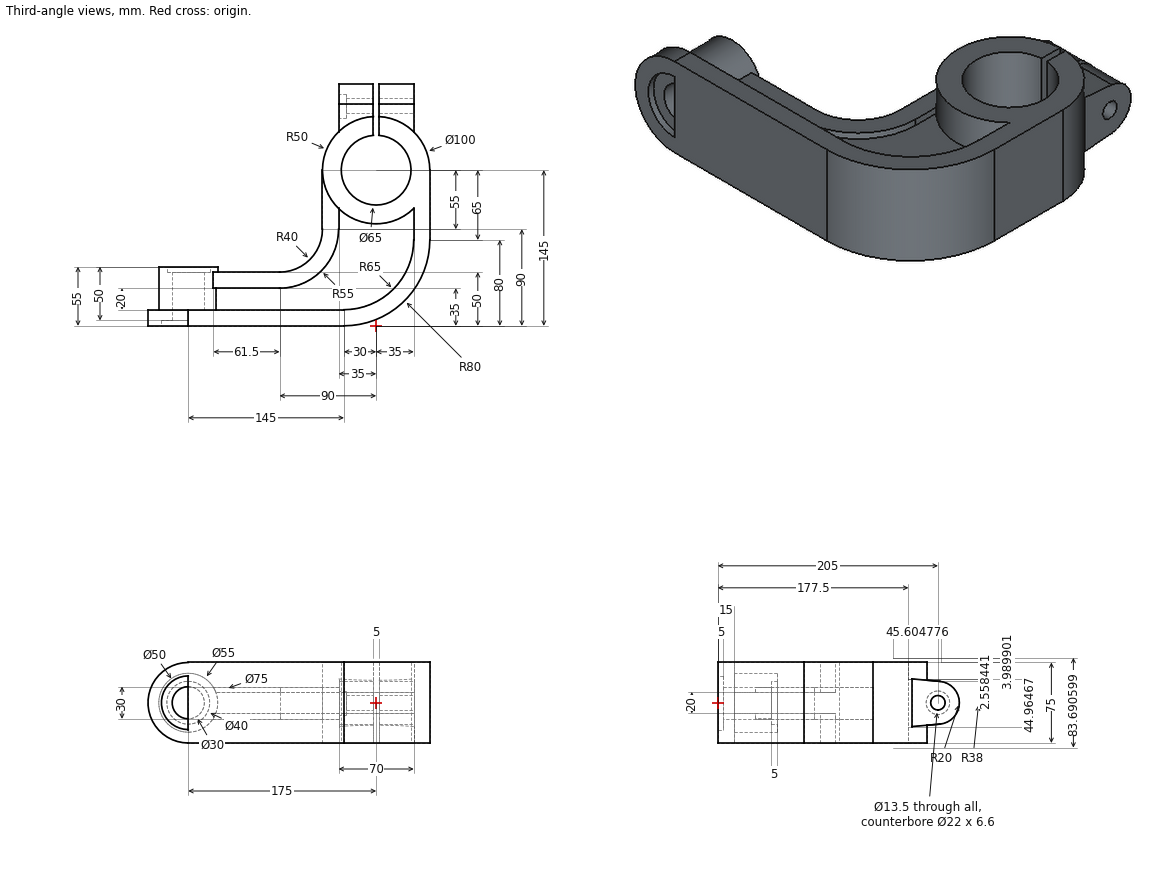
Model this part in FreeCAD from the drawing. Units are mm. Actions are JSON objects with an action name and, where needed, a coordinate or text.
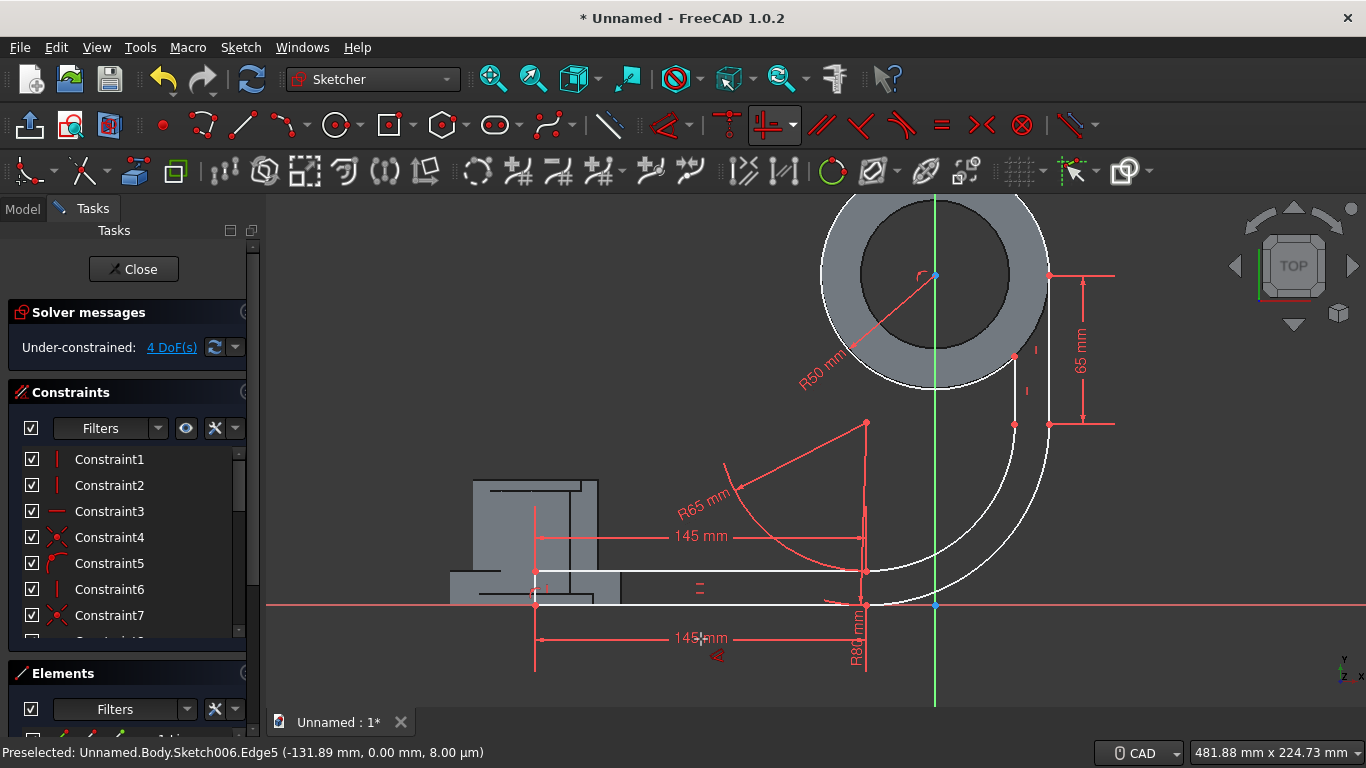
{"action": "left_click", "coordinate": [1049, 424]}
{"action": "left_click", "coordinate": [1083, 515]}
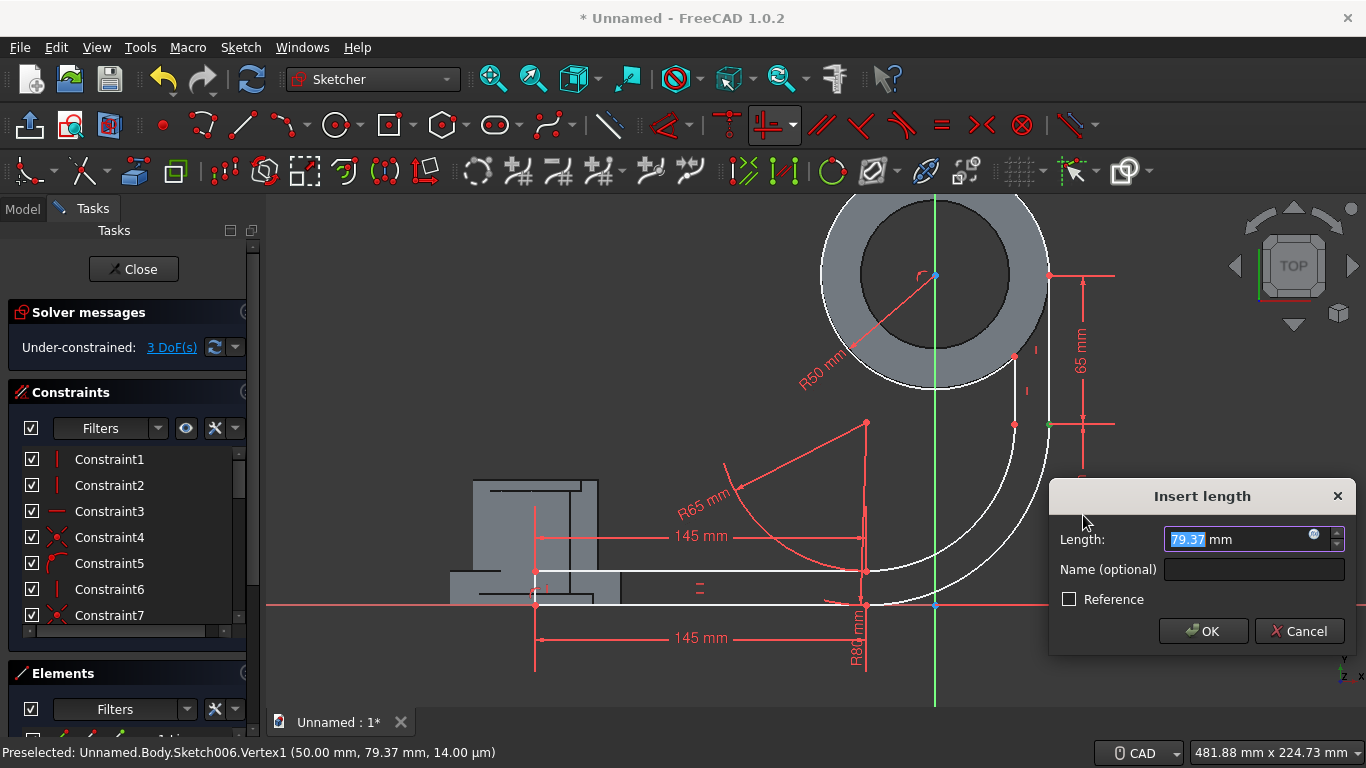
{"action": "type", "text": "80"}
{"action": "key", "text": "Return"}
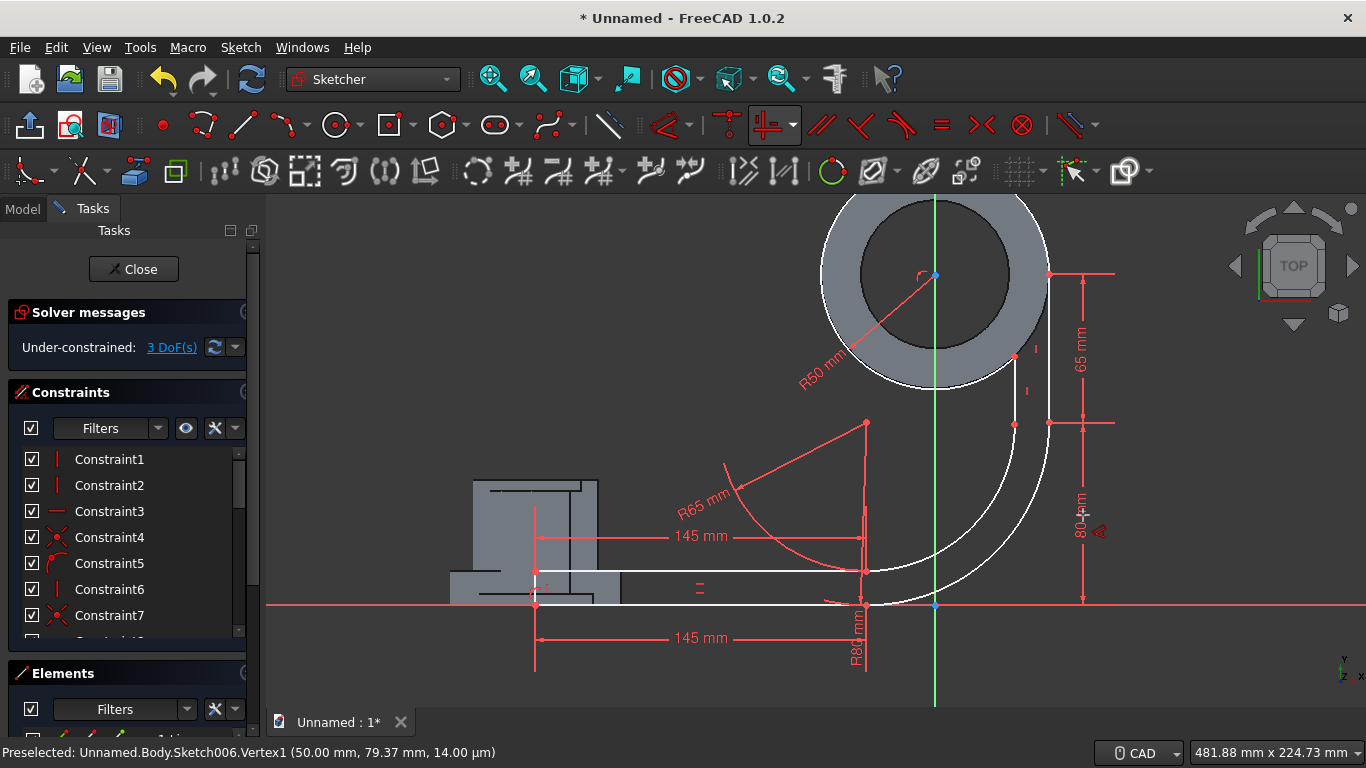
{"action": "left_click", "coordinate": [1015, 424]}
{"action": "left_click", "coordinate": [1049, 556]}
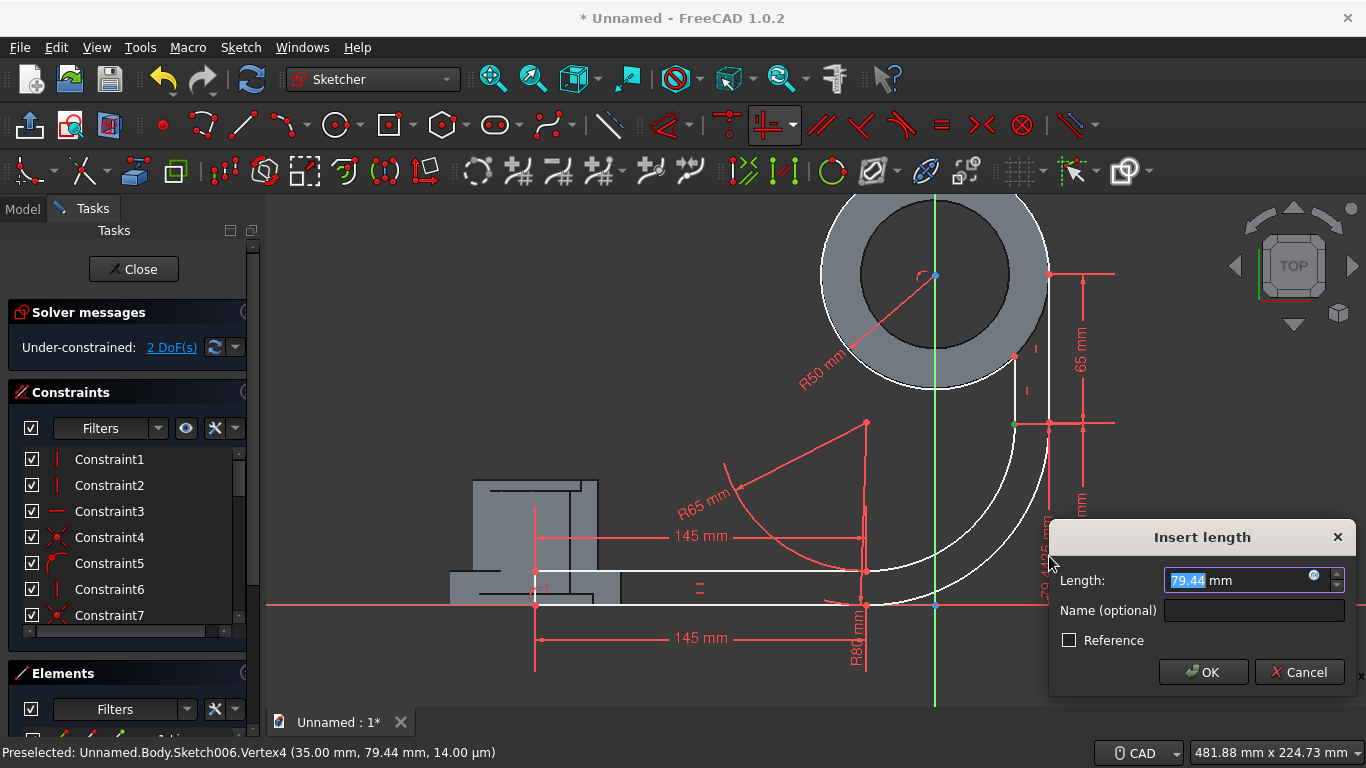
{"action": "type", "text": "80"}
{"action": "key", "text": "Return"}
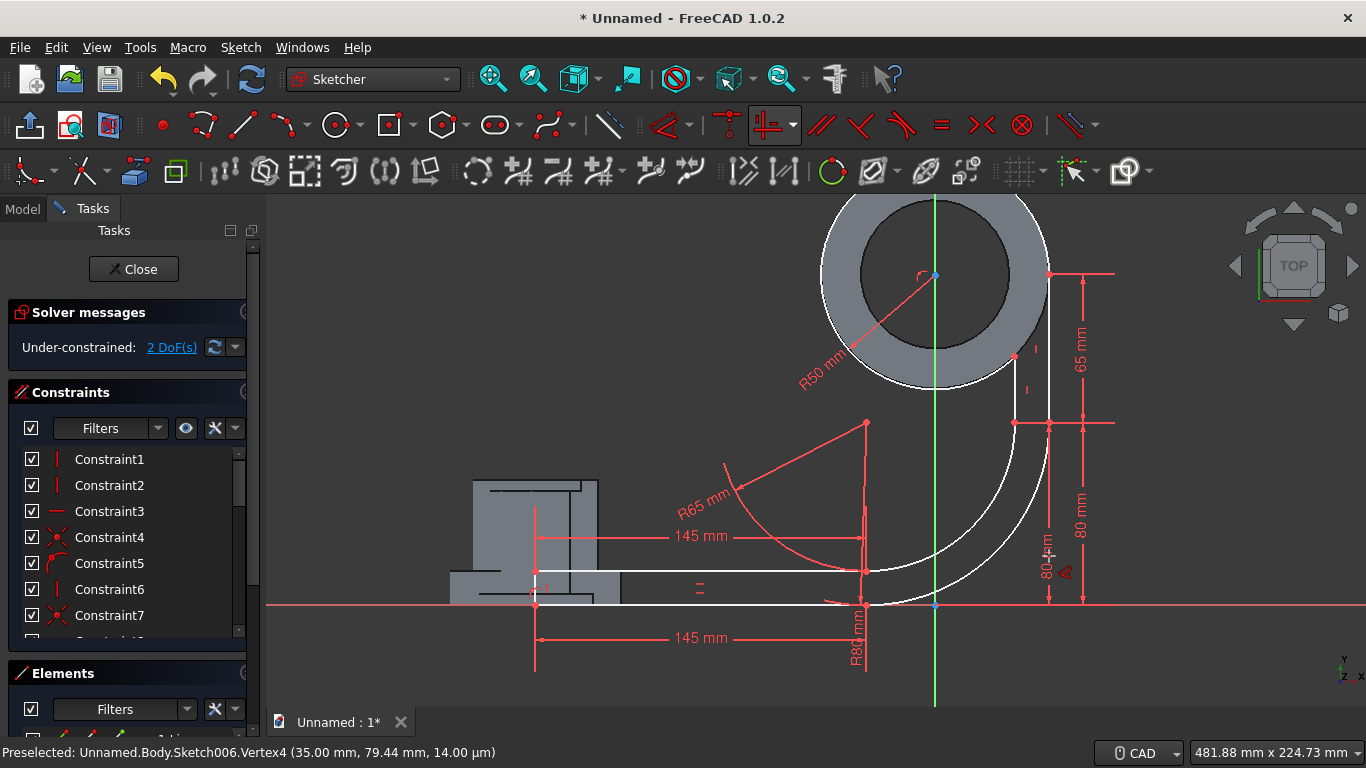
{"action": "left_click", "coordinate": [866, 571]}
{"action": "left_click", "coordinate": [901, 537]}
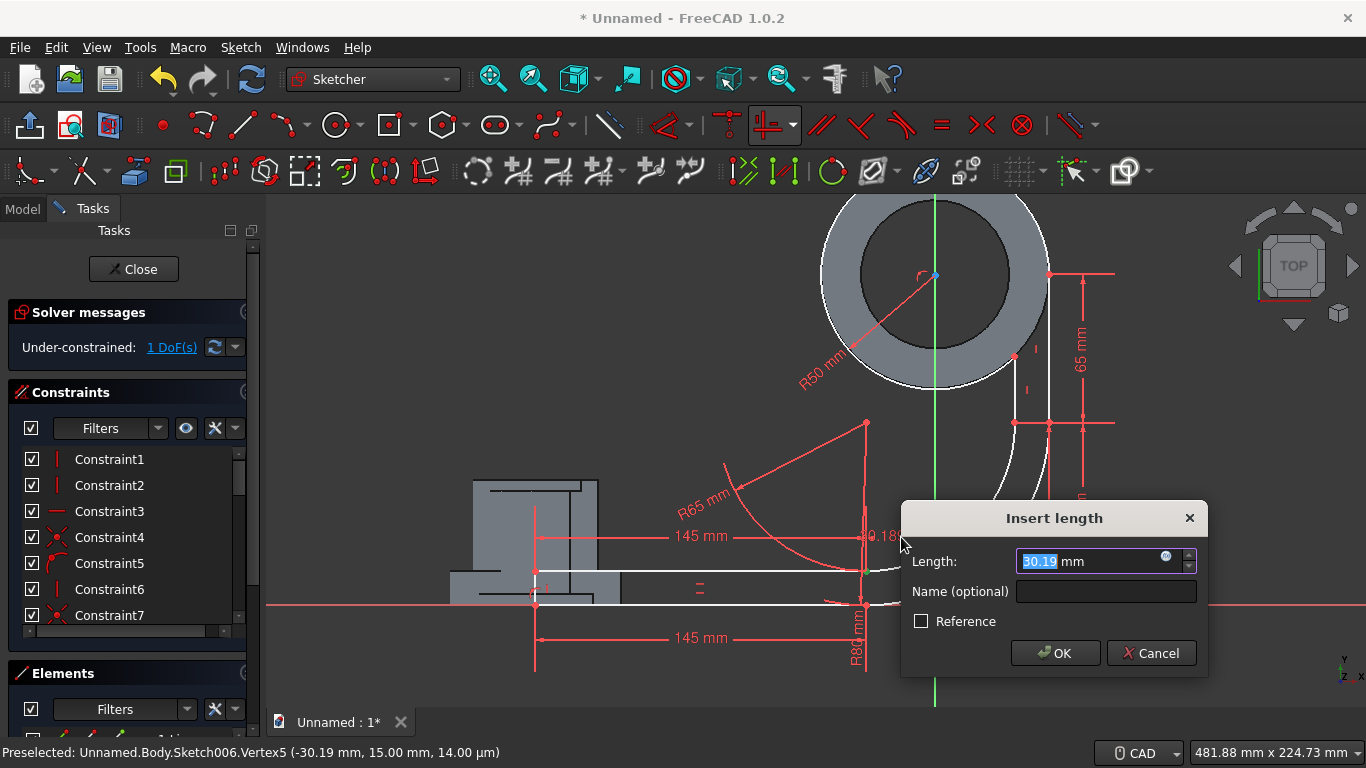
{"action": "type", "text": "30"}
{"action": "key", "text": "Return"}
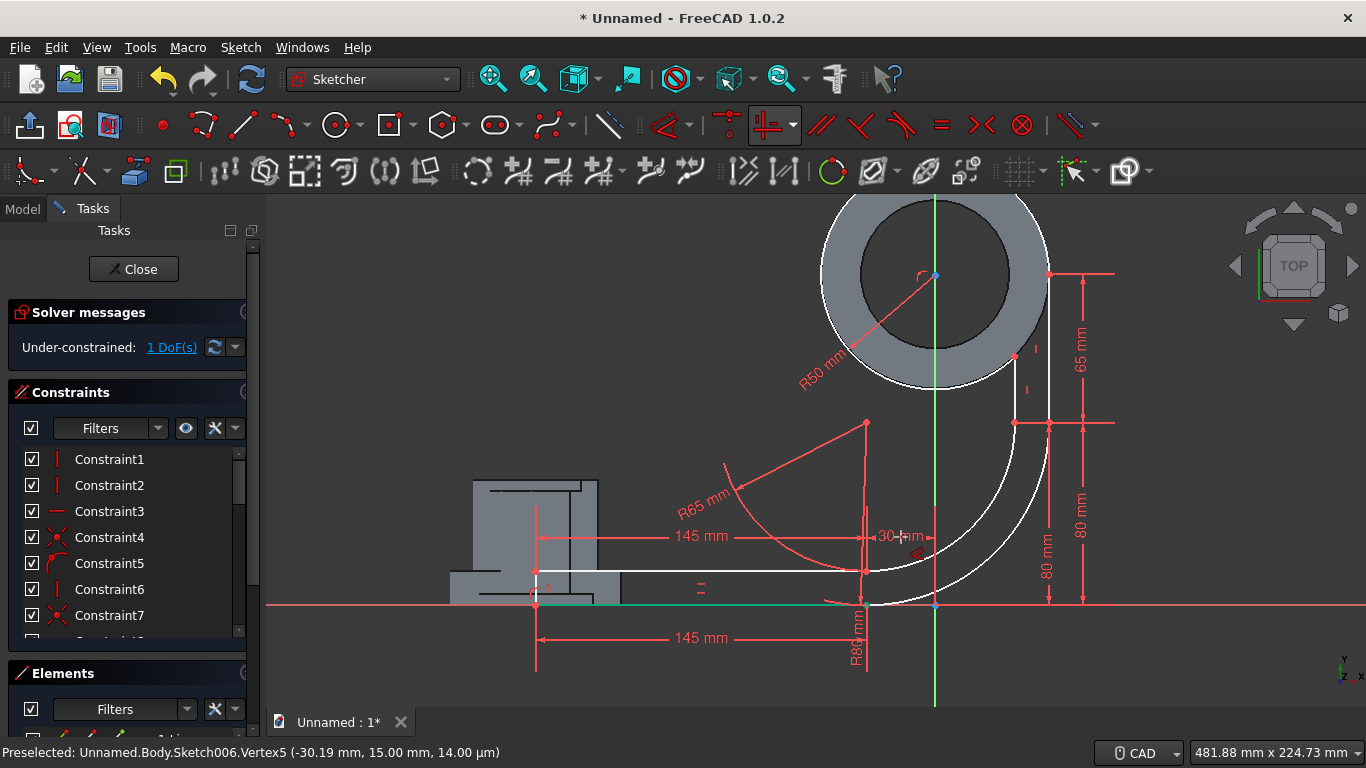
{"action": "left_click", "coordinate": [935, 275]}
{"action": "left_click", "coordinate": [969, 440]}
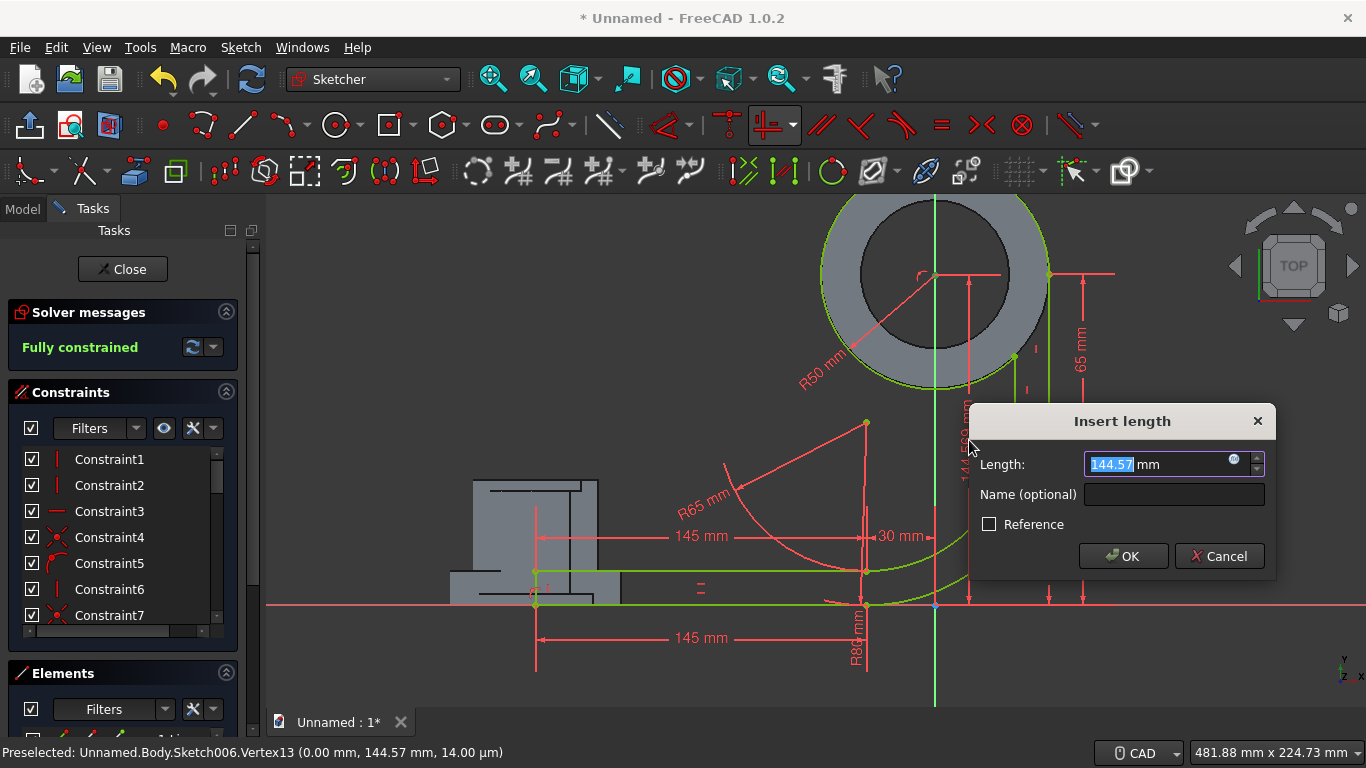
{"action": "type", "text": "145"}
{"action": "key", "text": "Return"}
{"action": "key", "text": "Escape"}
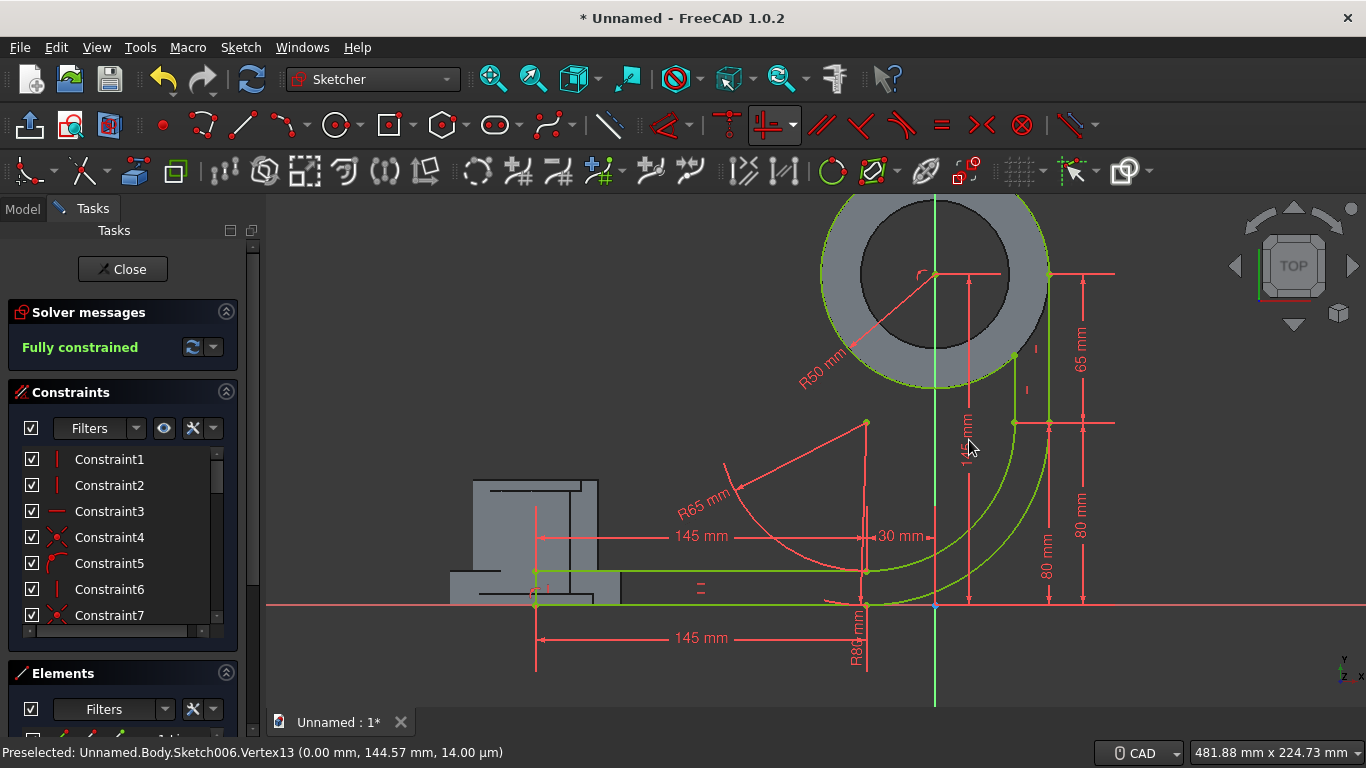
{"action": "left_click", "coordinate": [123, 269]}